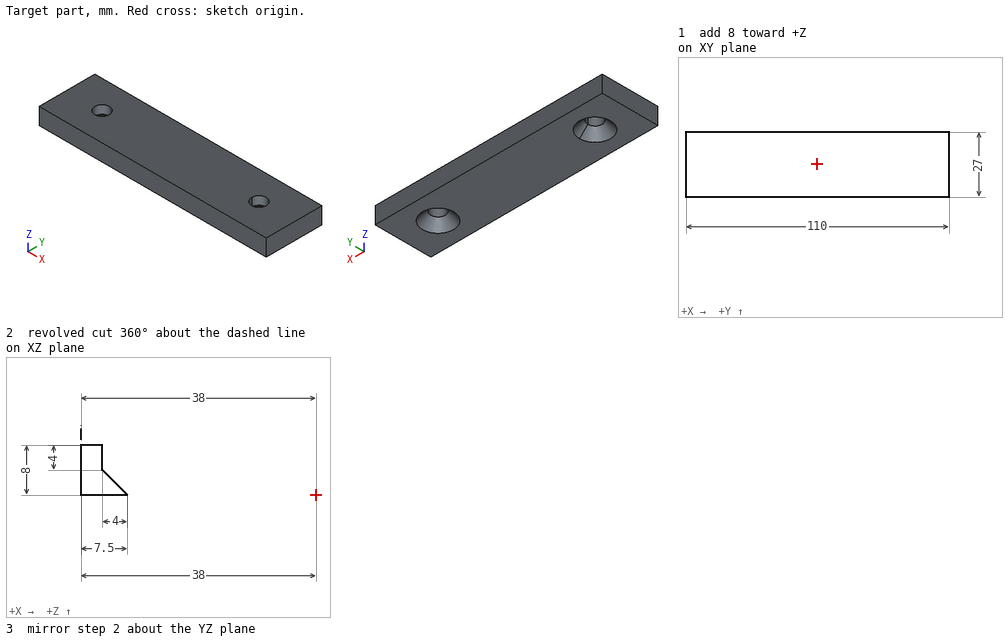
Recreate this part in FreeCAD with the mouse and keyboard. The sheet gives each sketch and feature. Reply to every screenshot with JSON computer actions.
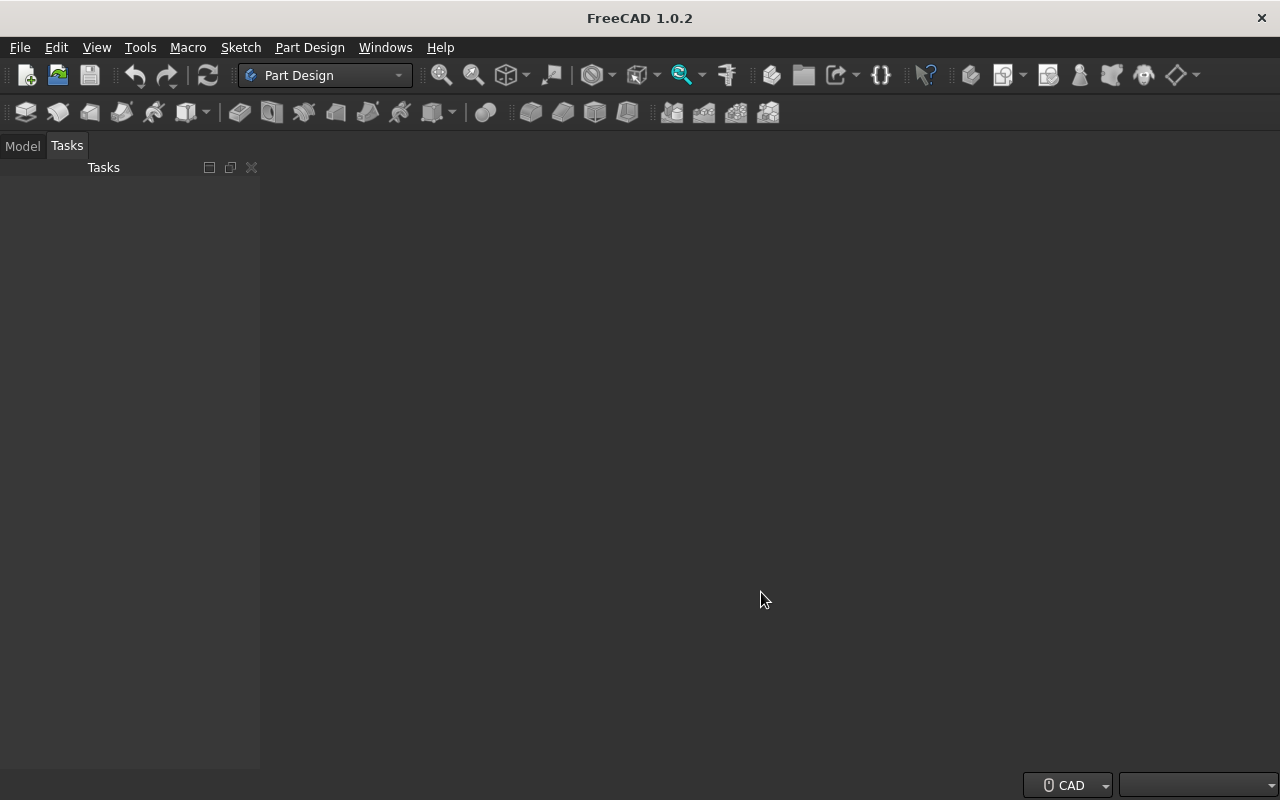
{"action": "left_click", "coordinate": [26, 76]}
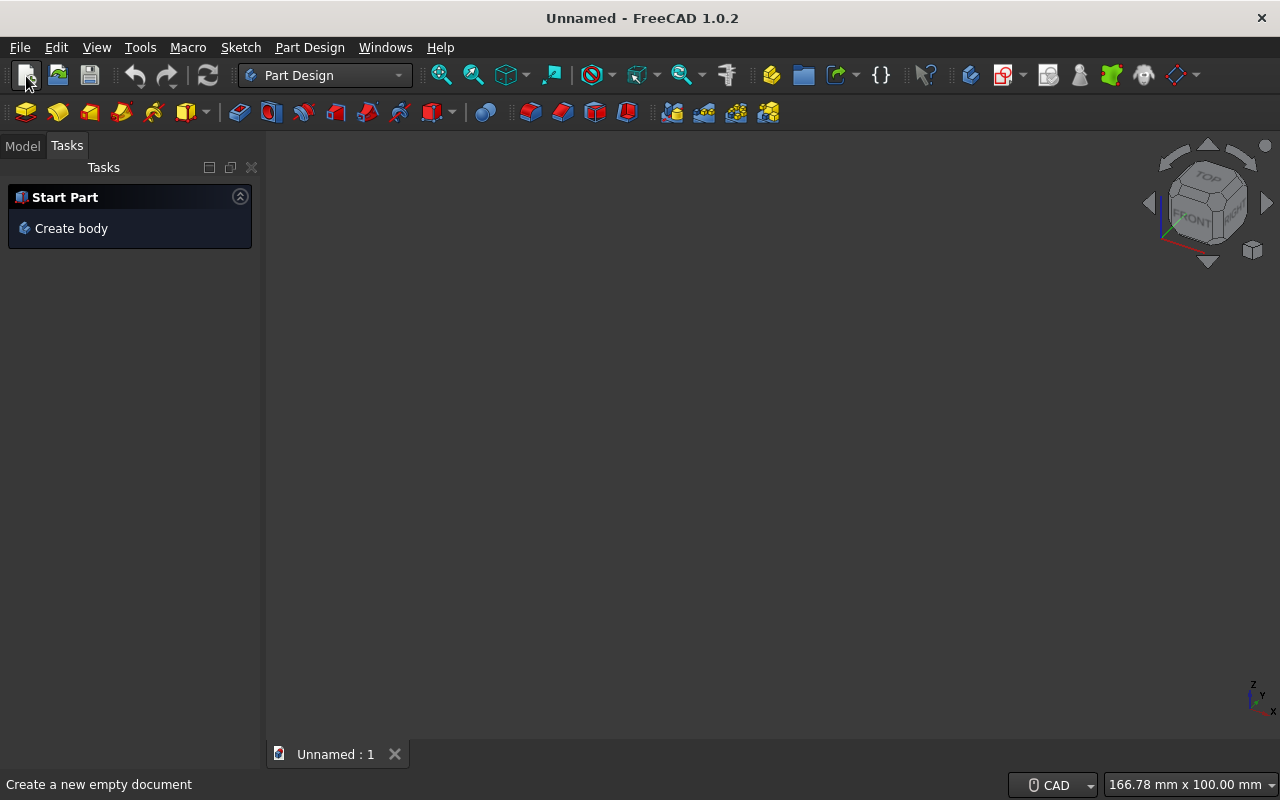
{"action": "left_click", "coordinate": [1004, 76]}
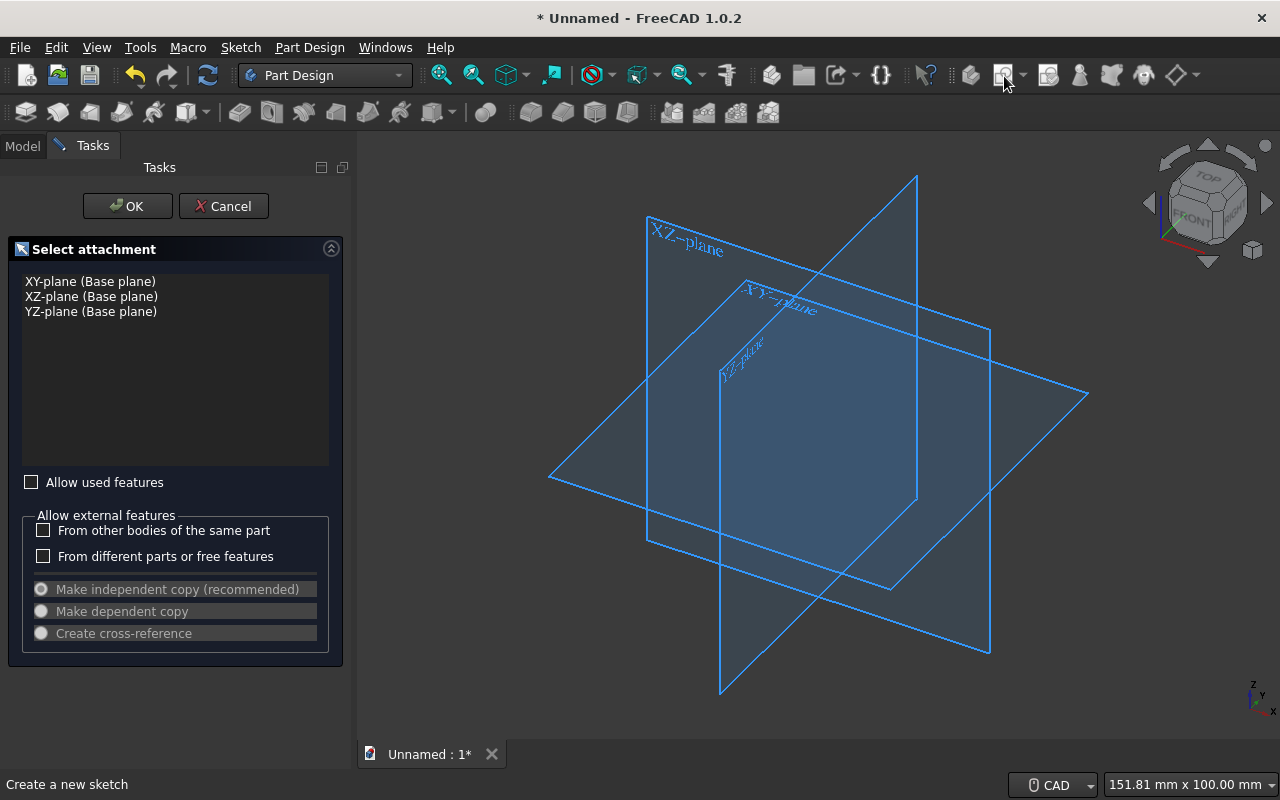
{"action": "left_click", "coordinate": [82, 282]}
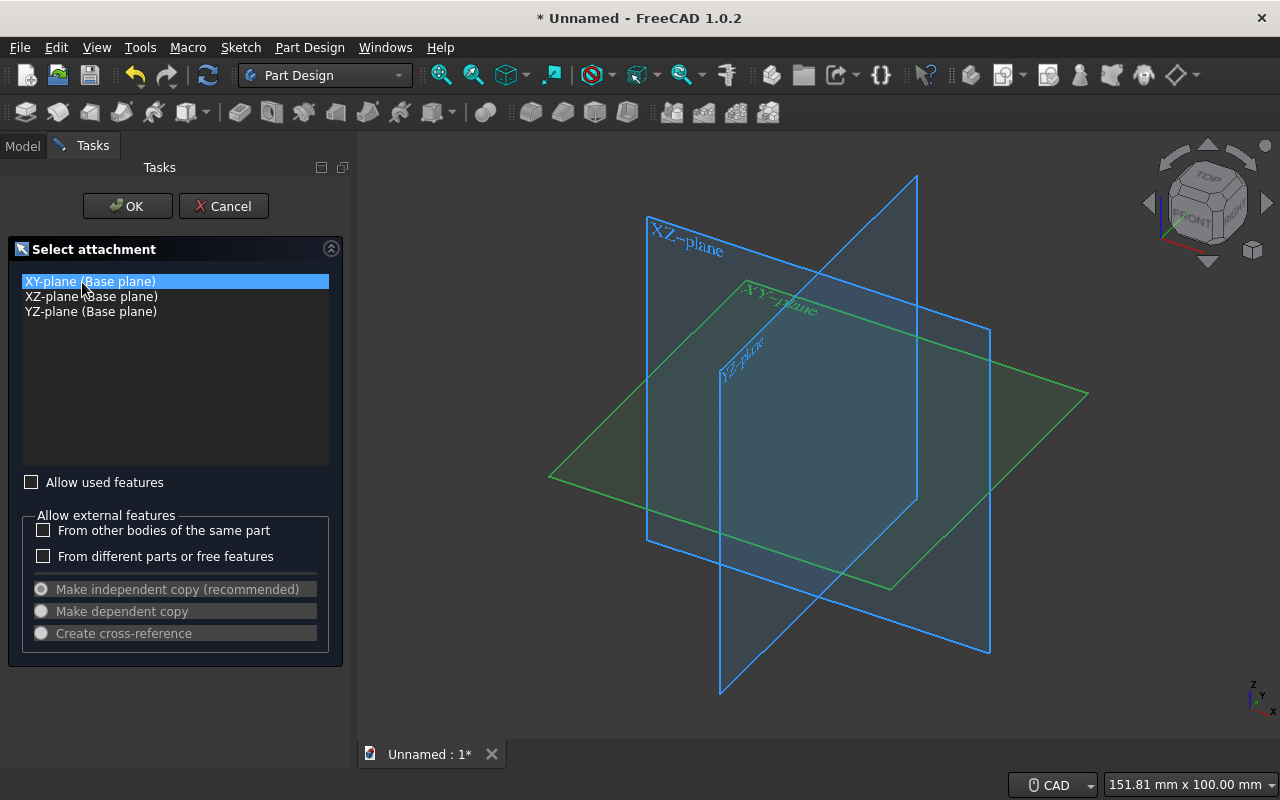
{"action": "left_click", "coordinate": [128, 206]}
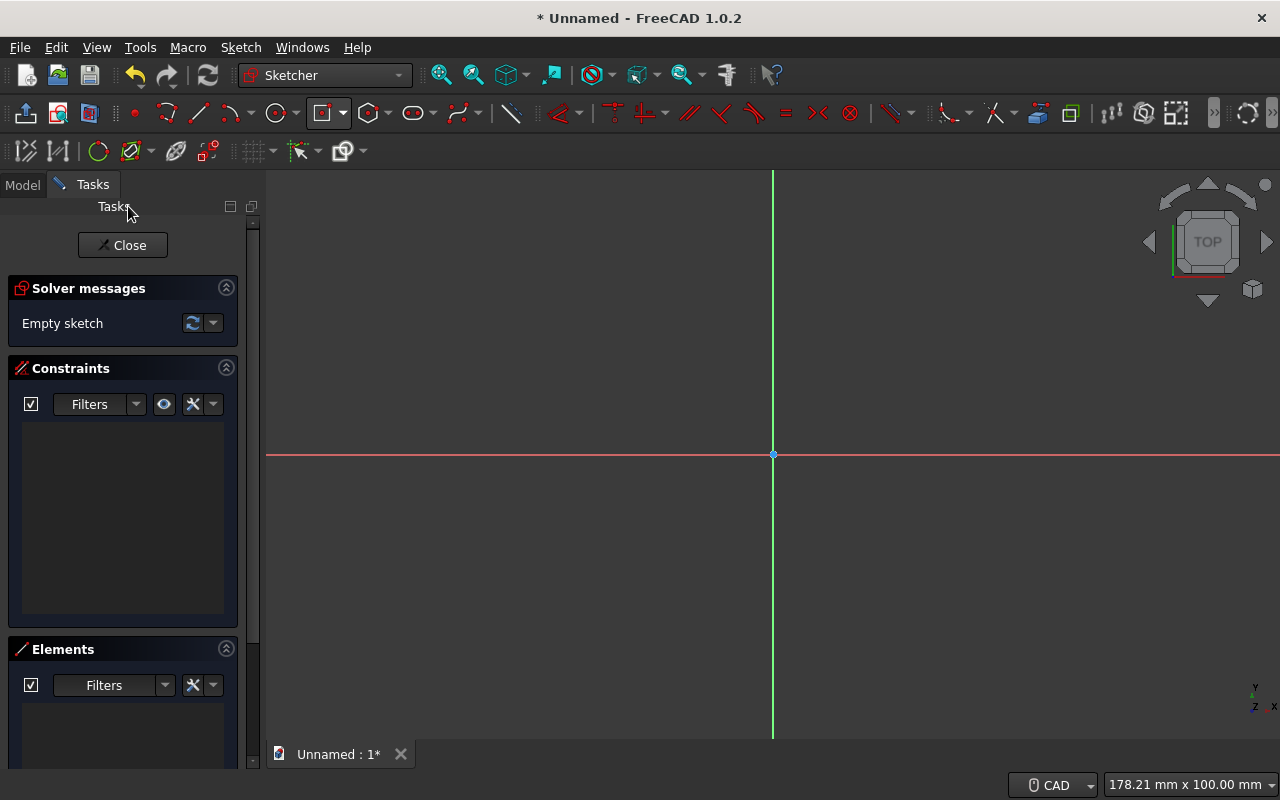
{"action": "left_click", "coordinate": [322, 114]}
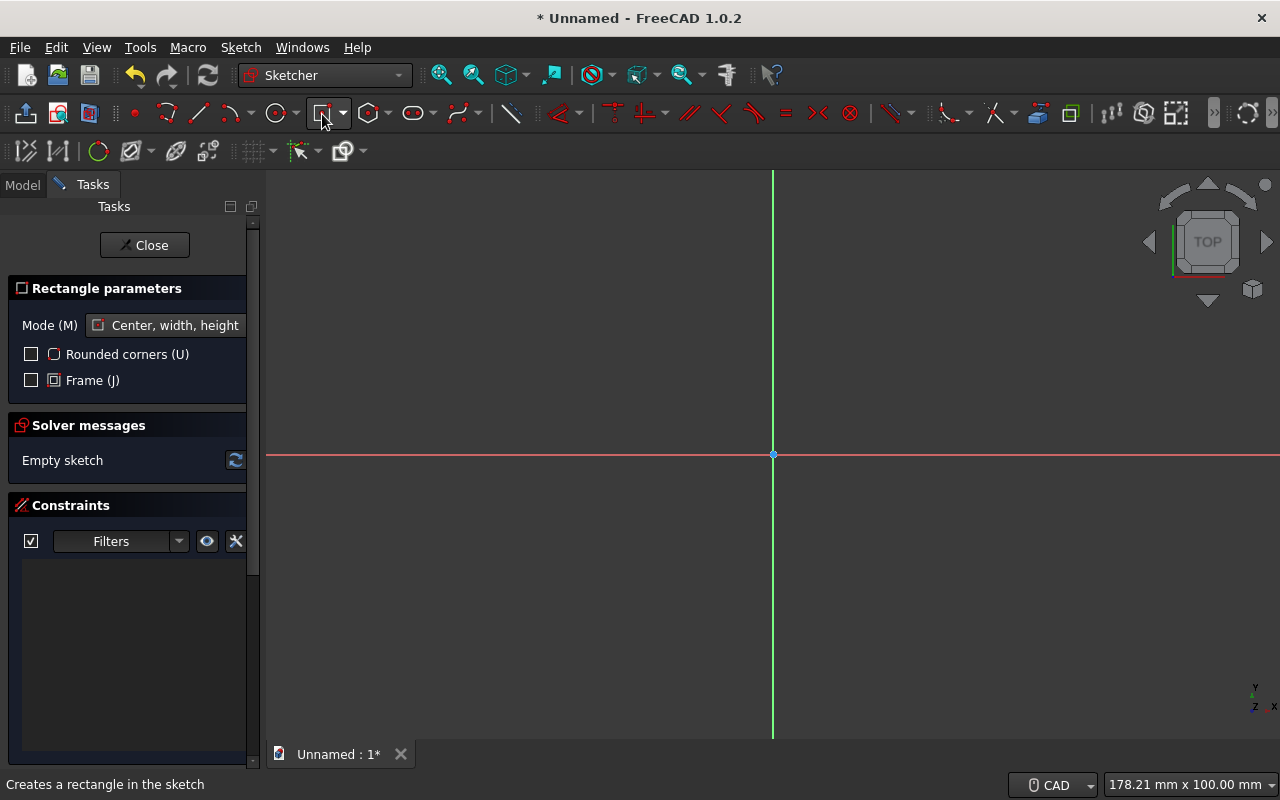
{"action": "left_click", "coordinate": [773, 454]}
{"action": "left_click", "coordinate": [1086, 378]}
{"action": "key", "text": "Escape"}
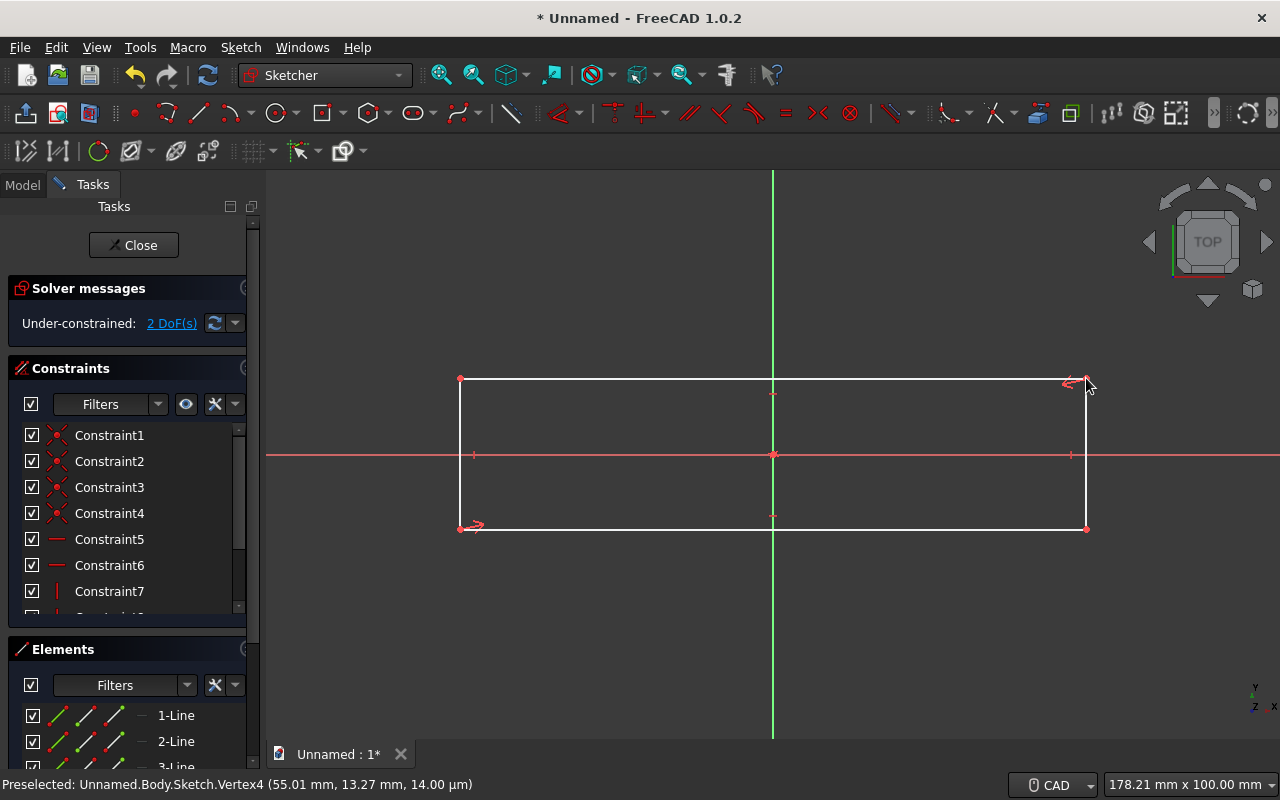
{"action": "left_click", "coordinate": [558, 114]}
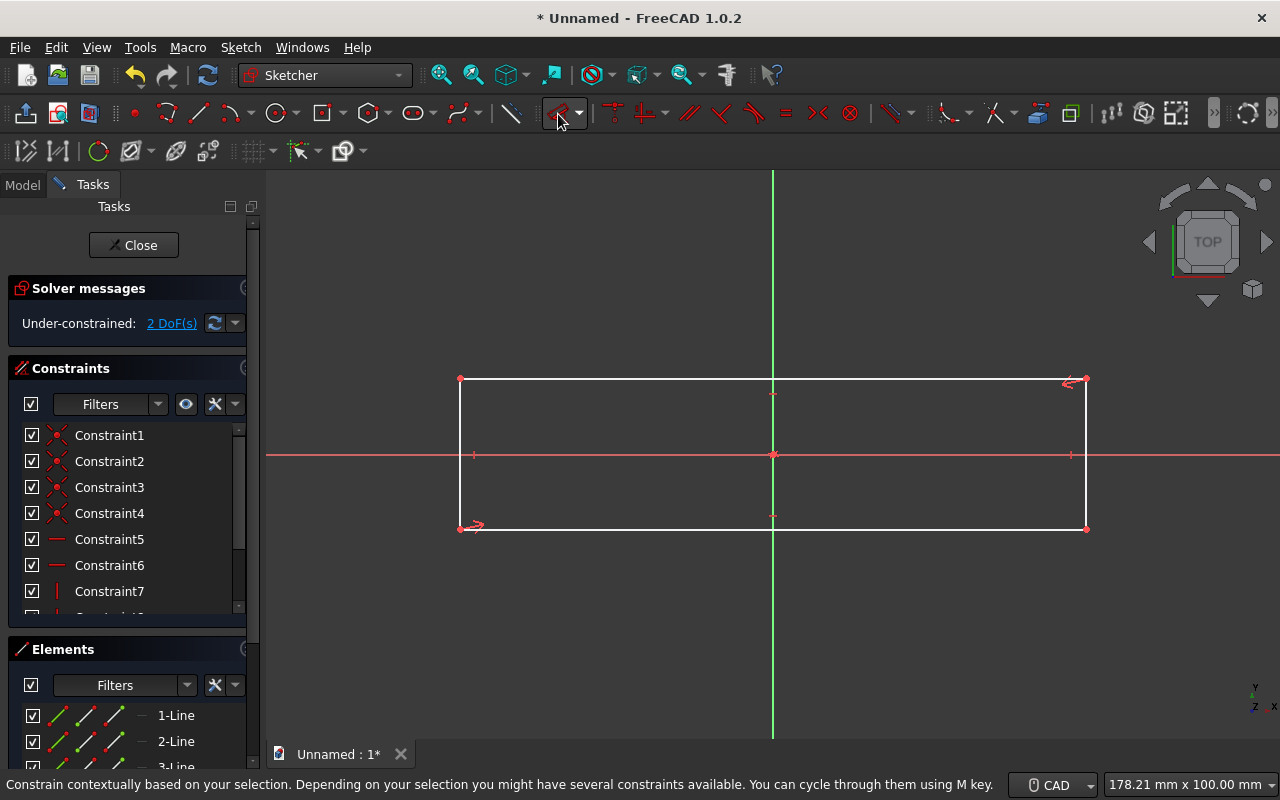
{"action": "left_click", "coordinate": [1086, 485]}
{"action": "left_click", "coordinate": [1052, 420]}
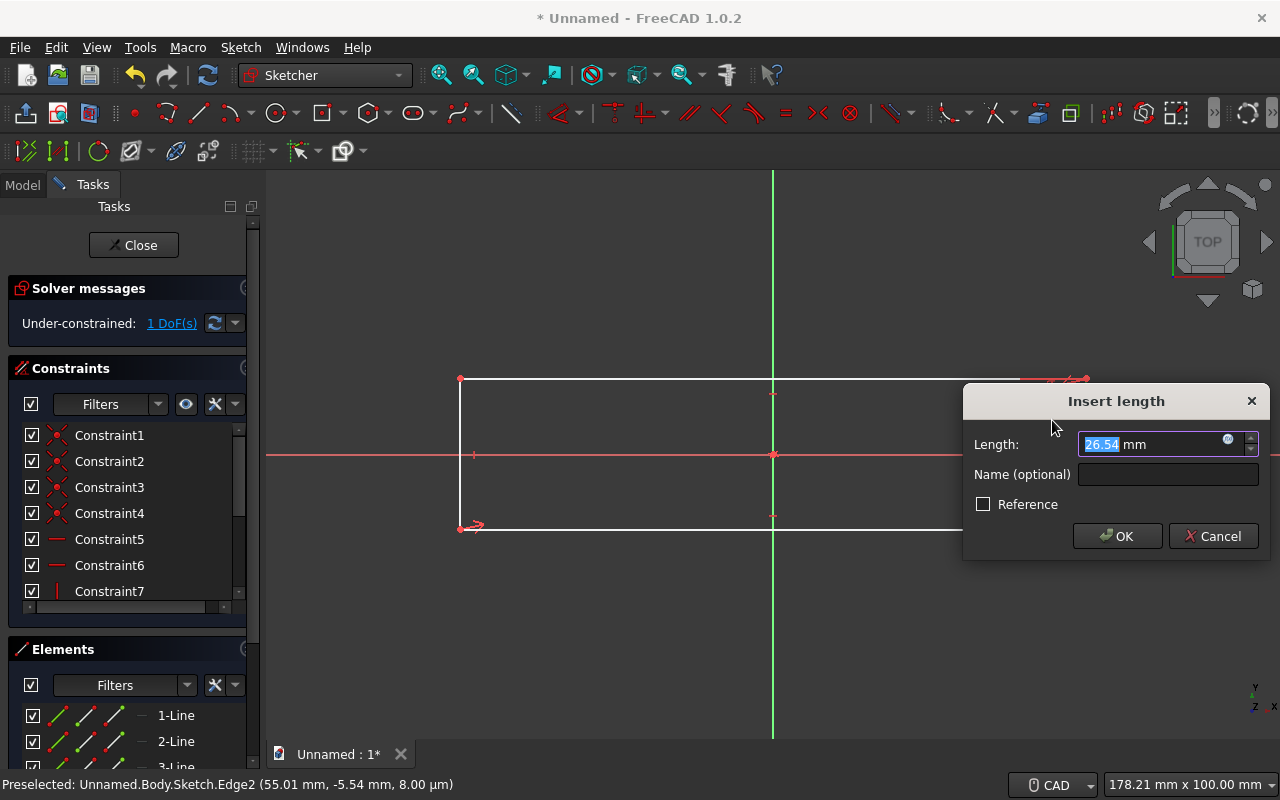
{"action": "type", "text": "27"}
{"action": "key", "text": "Return"}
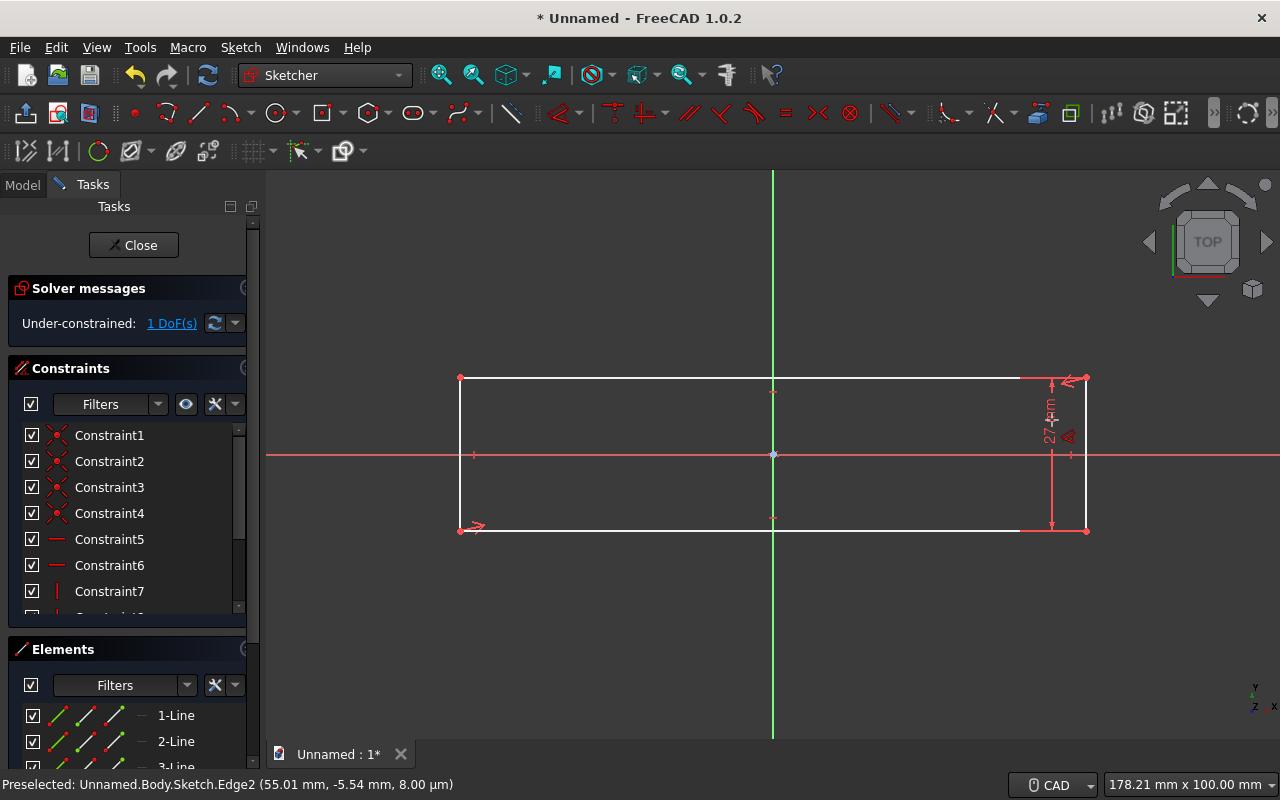
{"action": "left_click", "coordinate": [648, 531]}
{"action": "left_click", "coordinate": [629, 565]}